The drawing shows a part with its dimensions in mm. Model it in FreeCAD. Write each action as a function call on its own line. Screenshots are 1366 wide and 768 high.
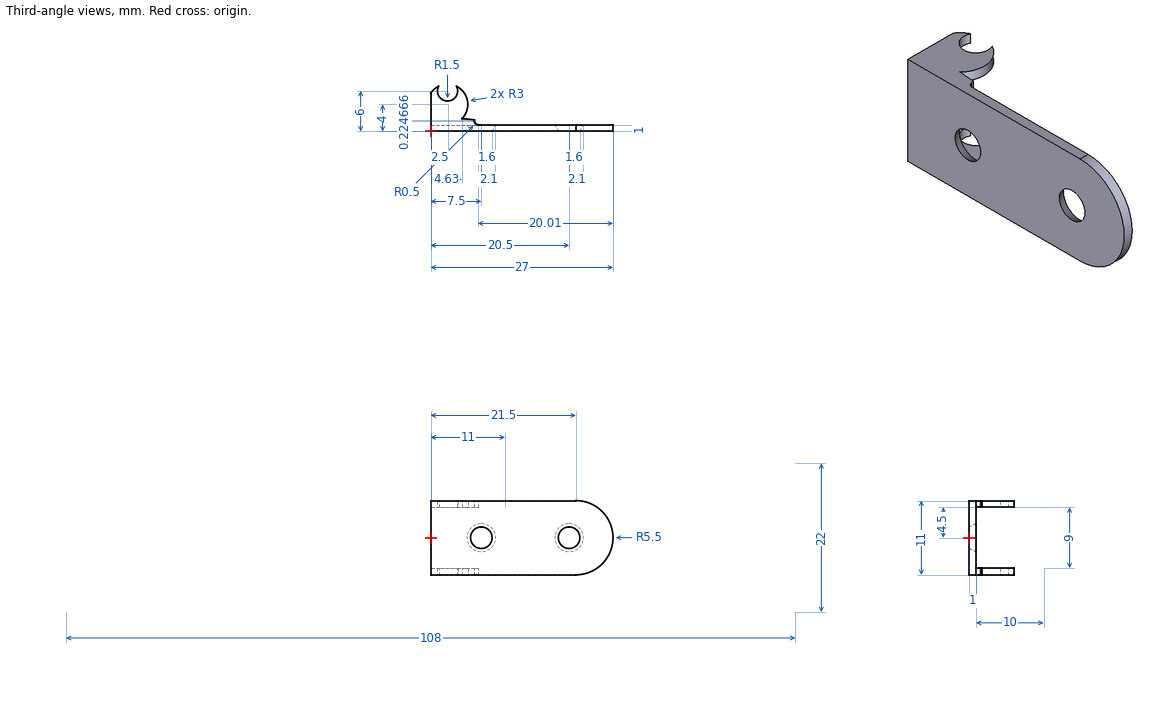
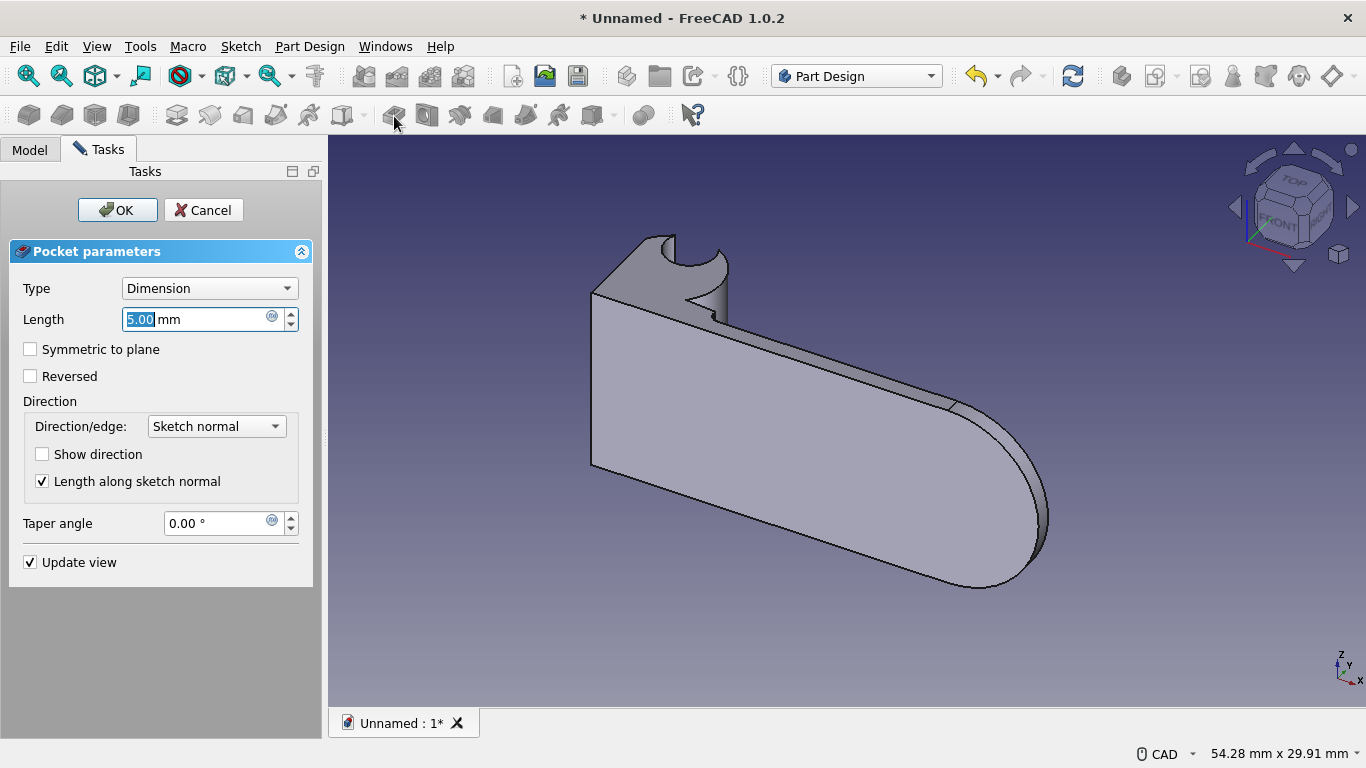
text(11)
key(Tab)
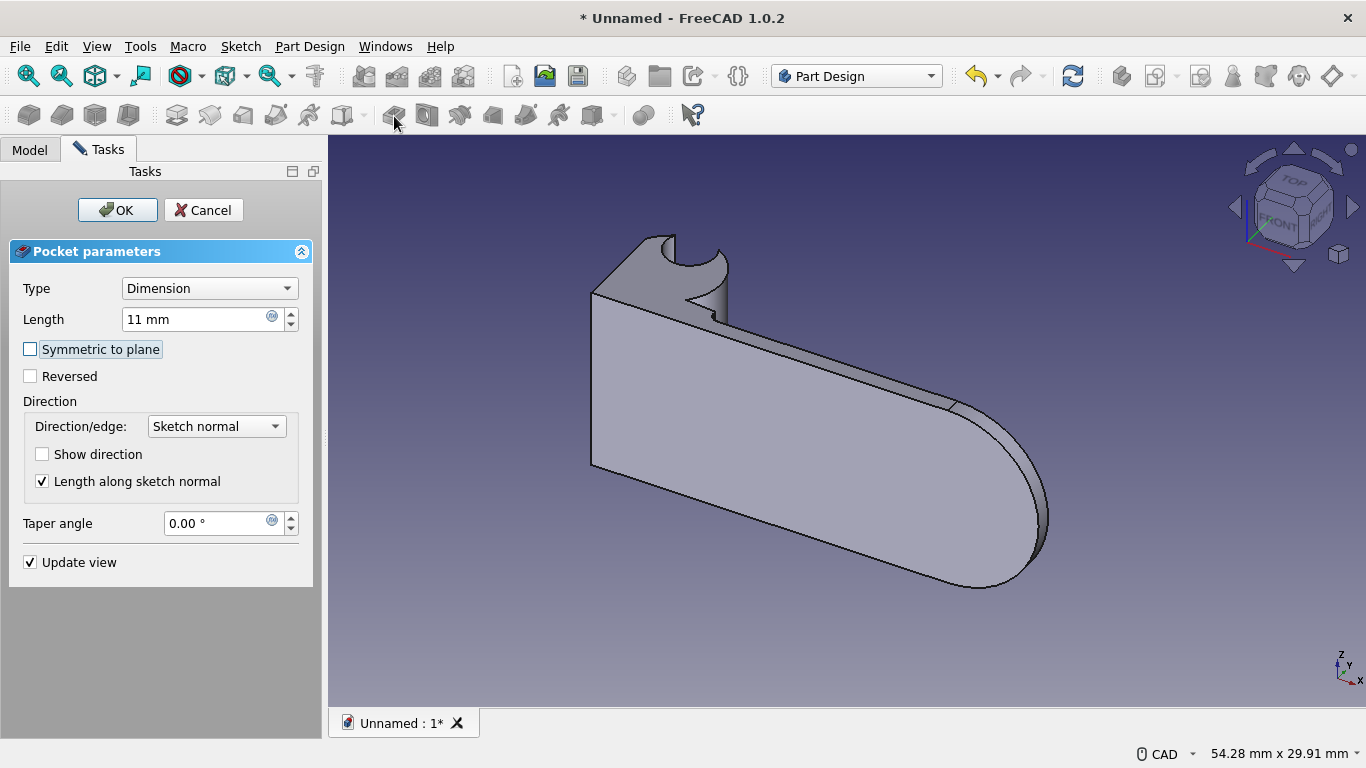
click(118, 210)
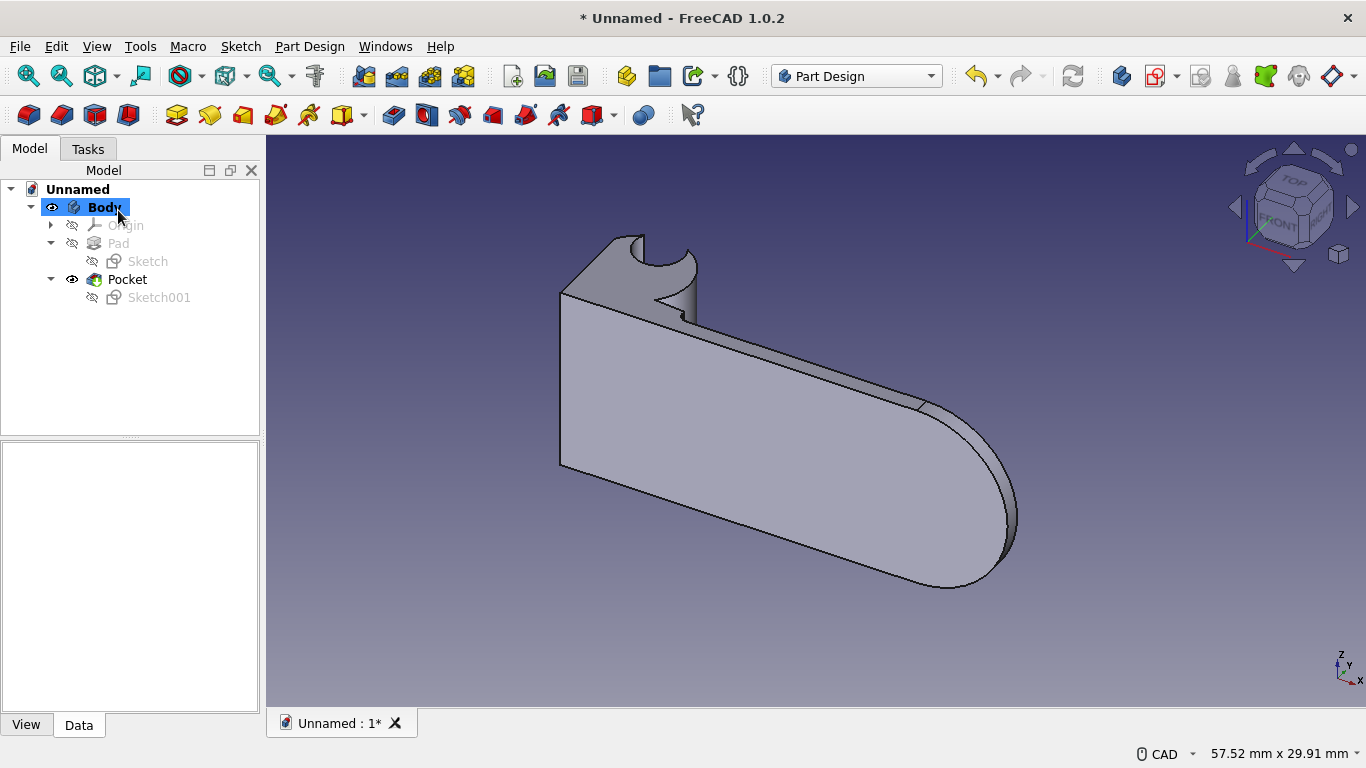
key(6)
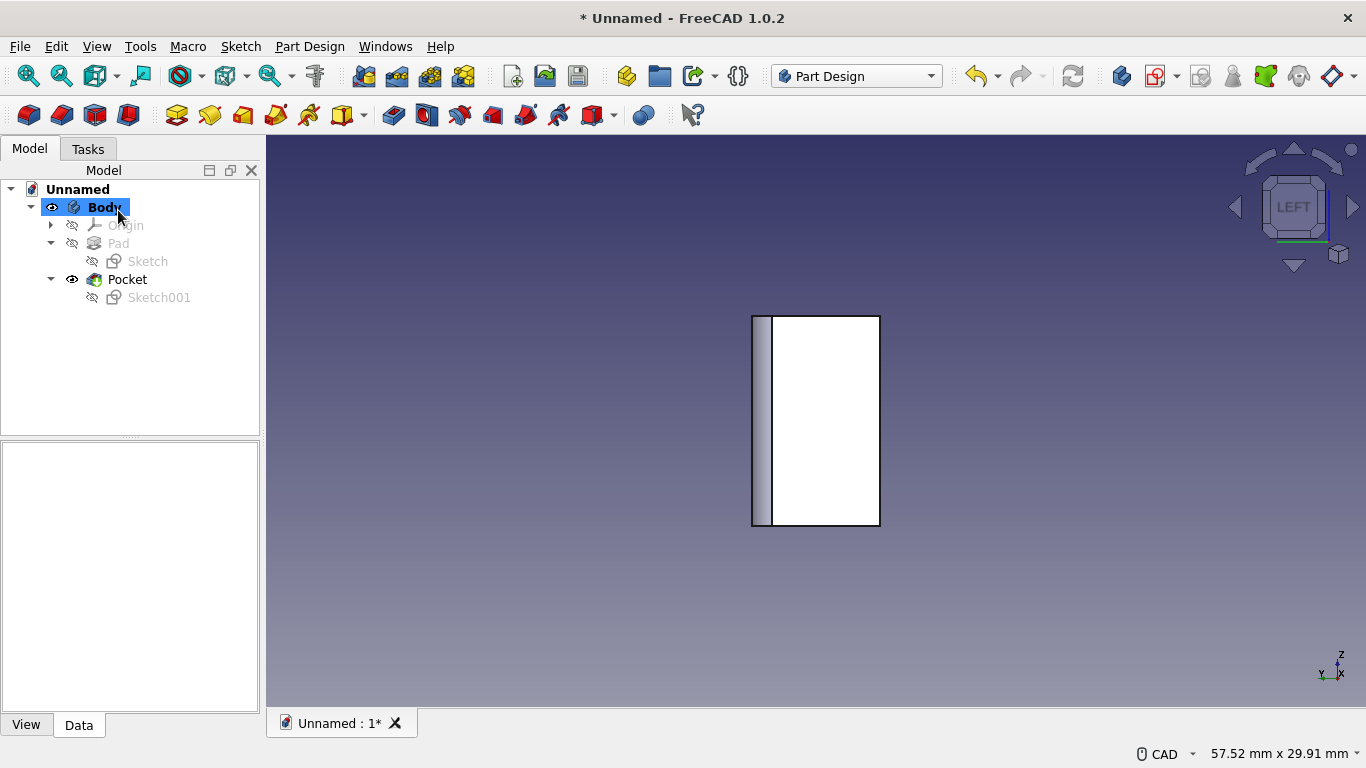
key(v)
key(f)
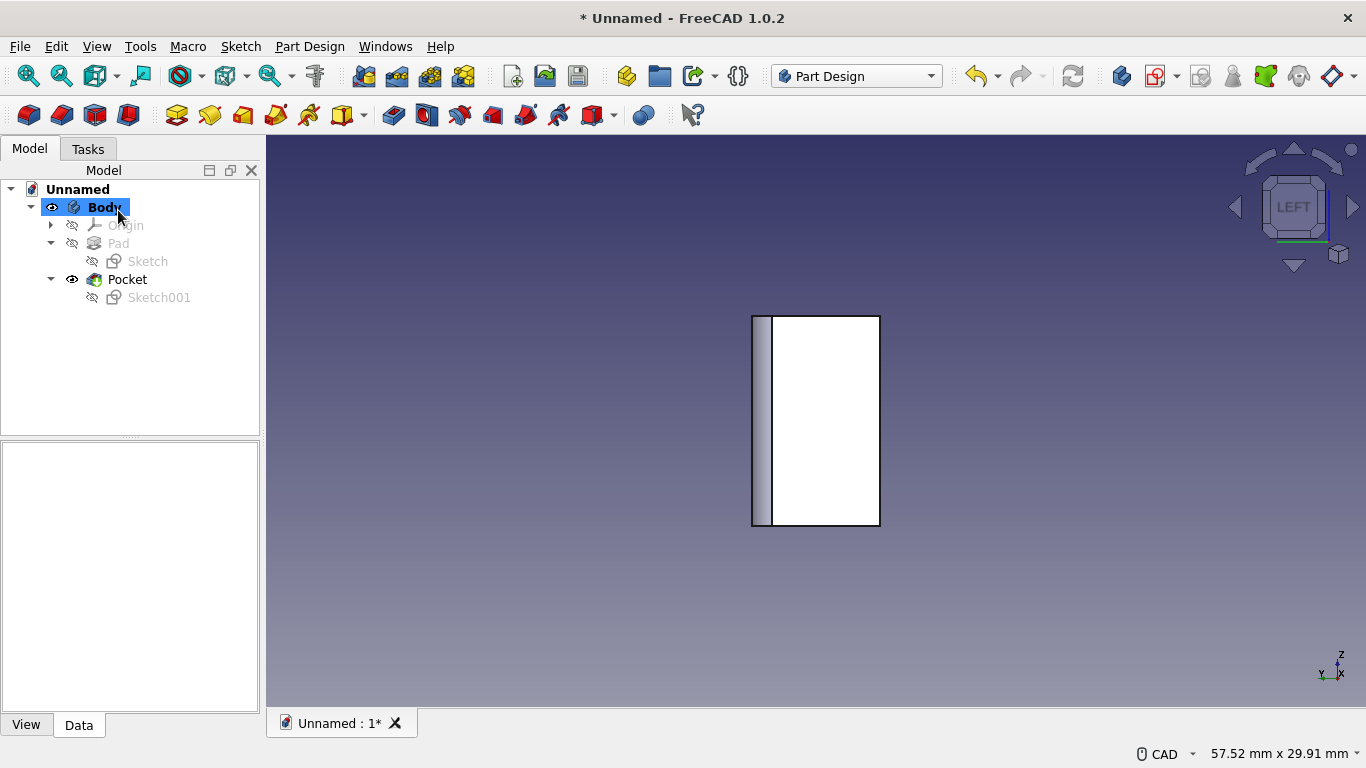
click(826, 390)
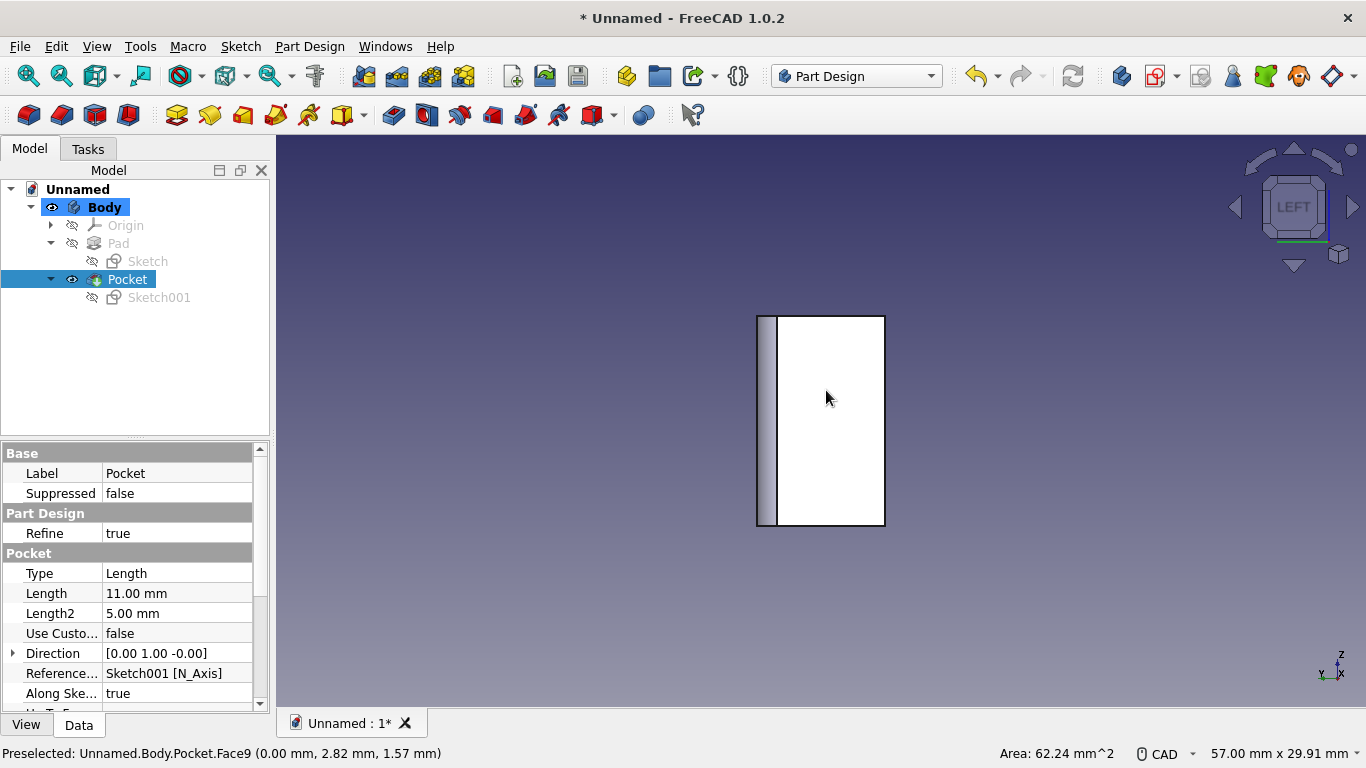
click(1154, 76)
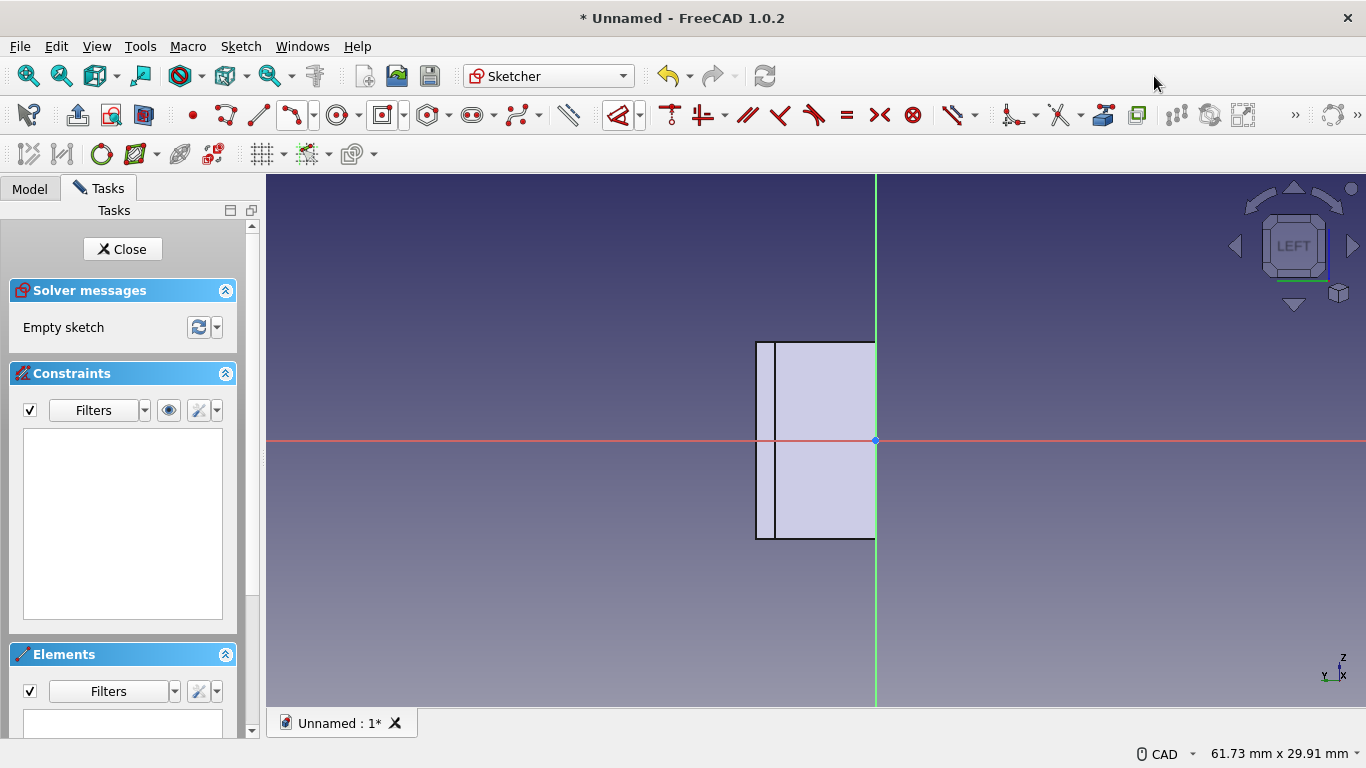
scroll(802, 440, up, 4)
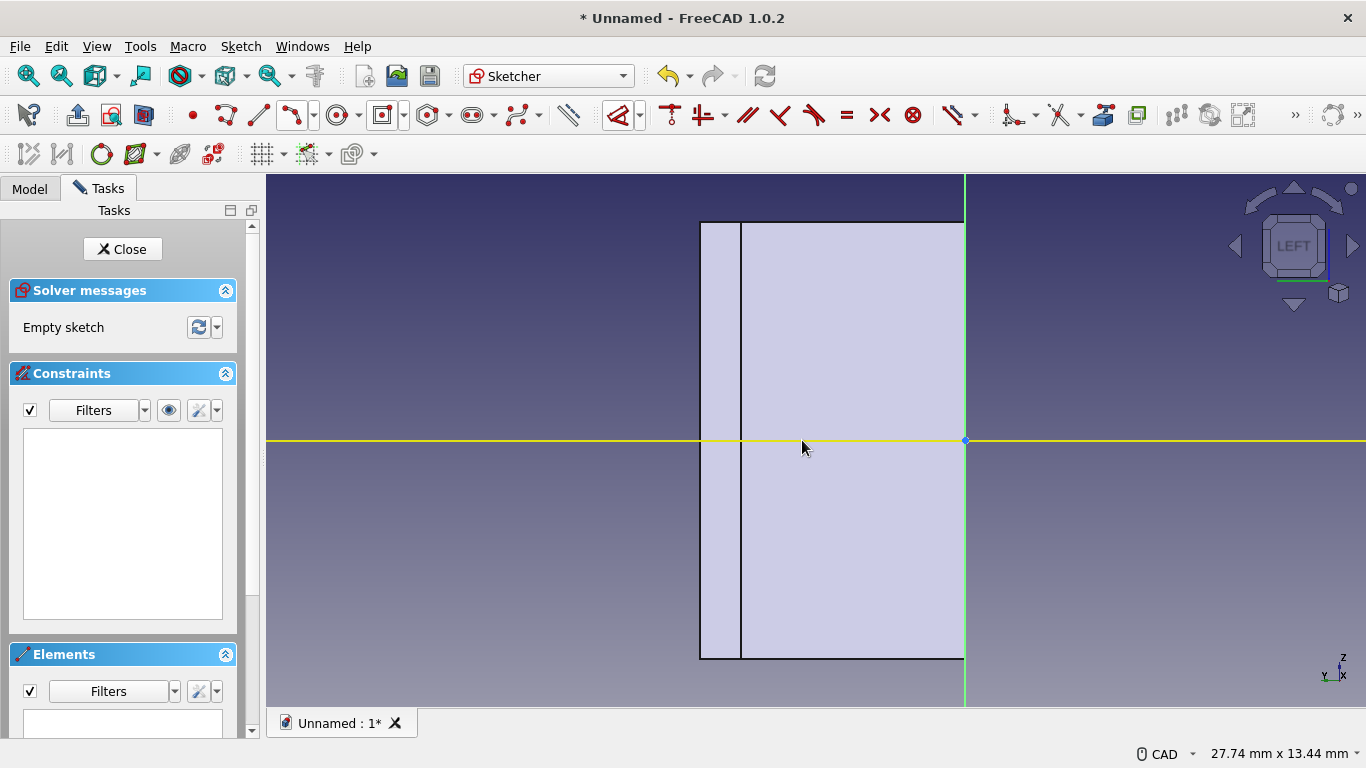
key(g)
key(r)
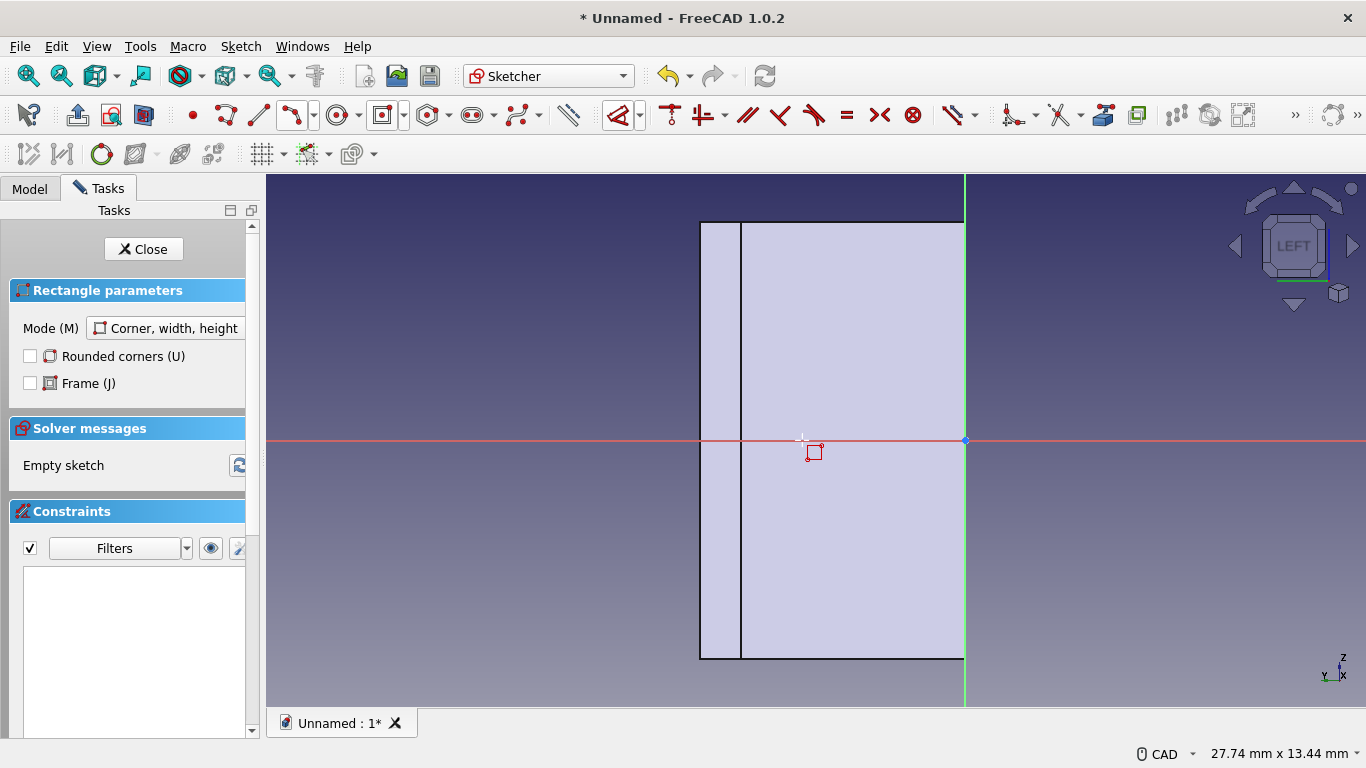
click(529, 262)
click(926, 619)
key(Escape)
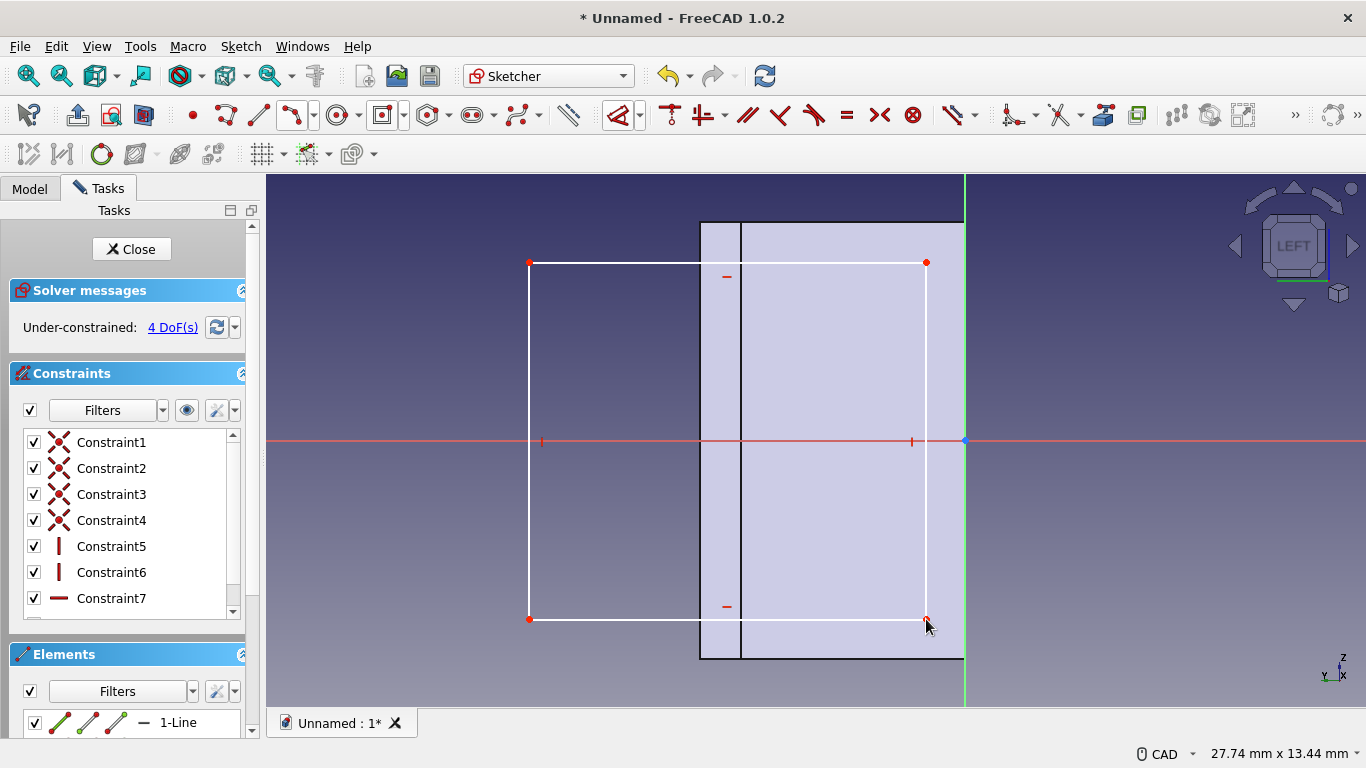
click(529, 370)